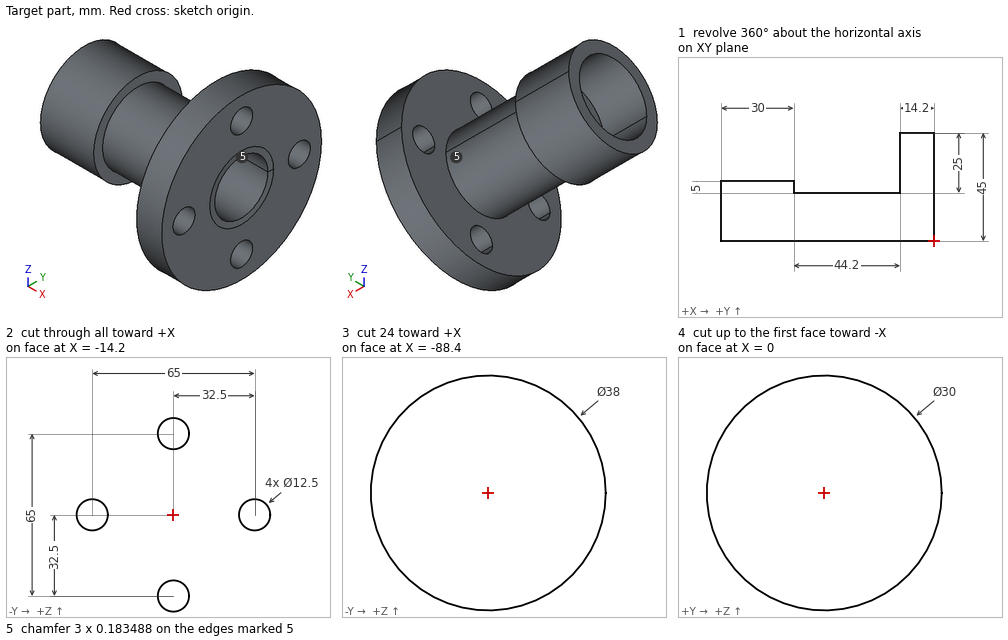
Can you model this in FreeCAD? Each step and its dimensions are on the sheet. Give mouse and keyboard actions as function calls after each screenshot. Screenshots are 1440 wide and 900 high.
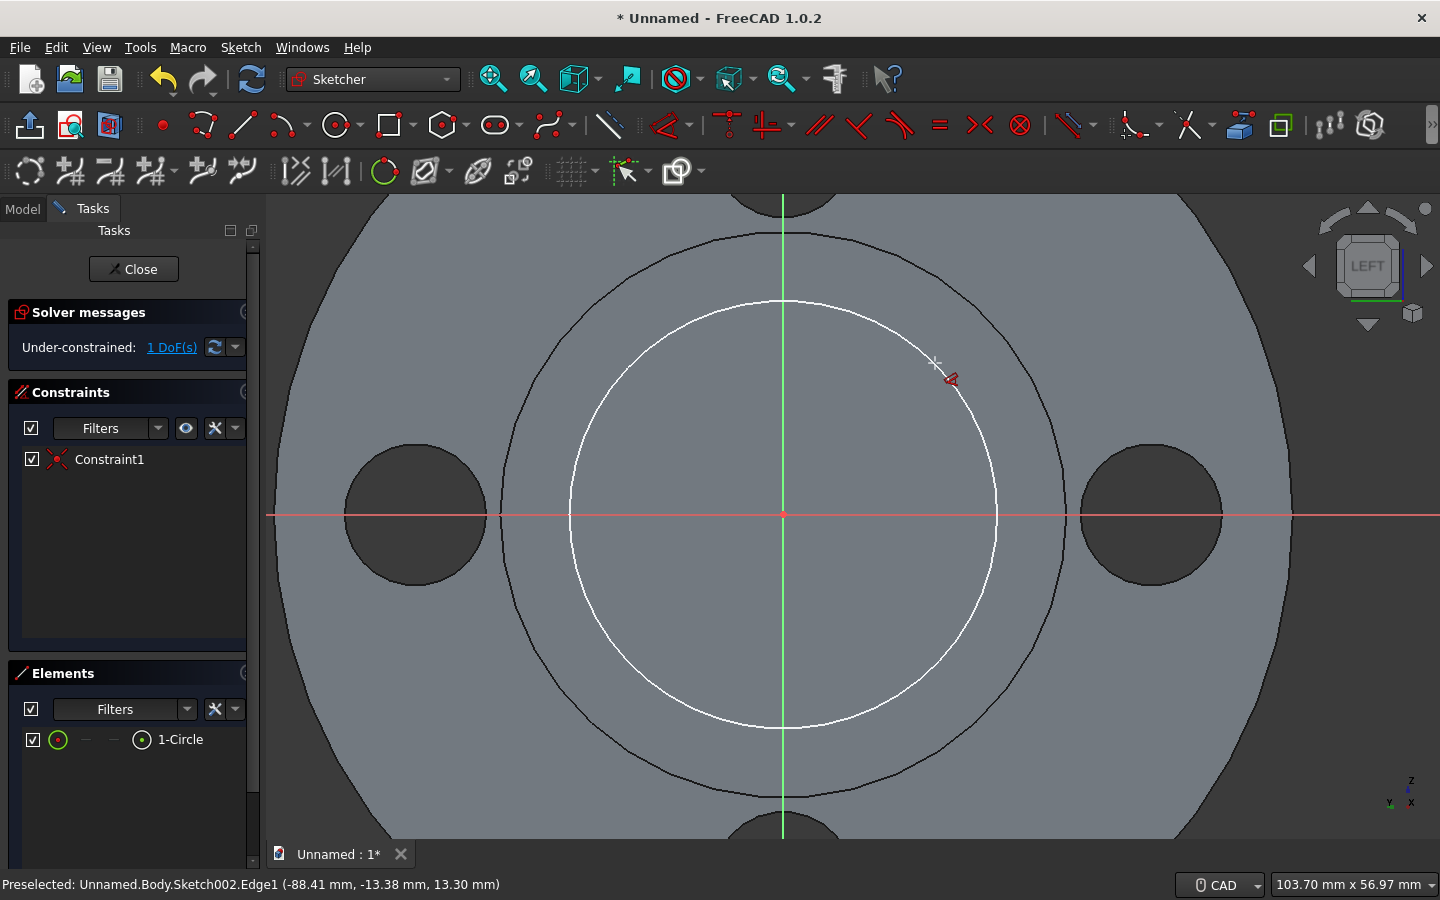
click(934, 363)
click(957, 340)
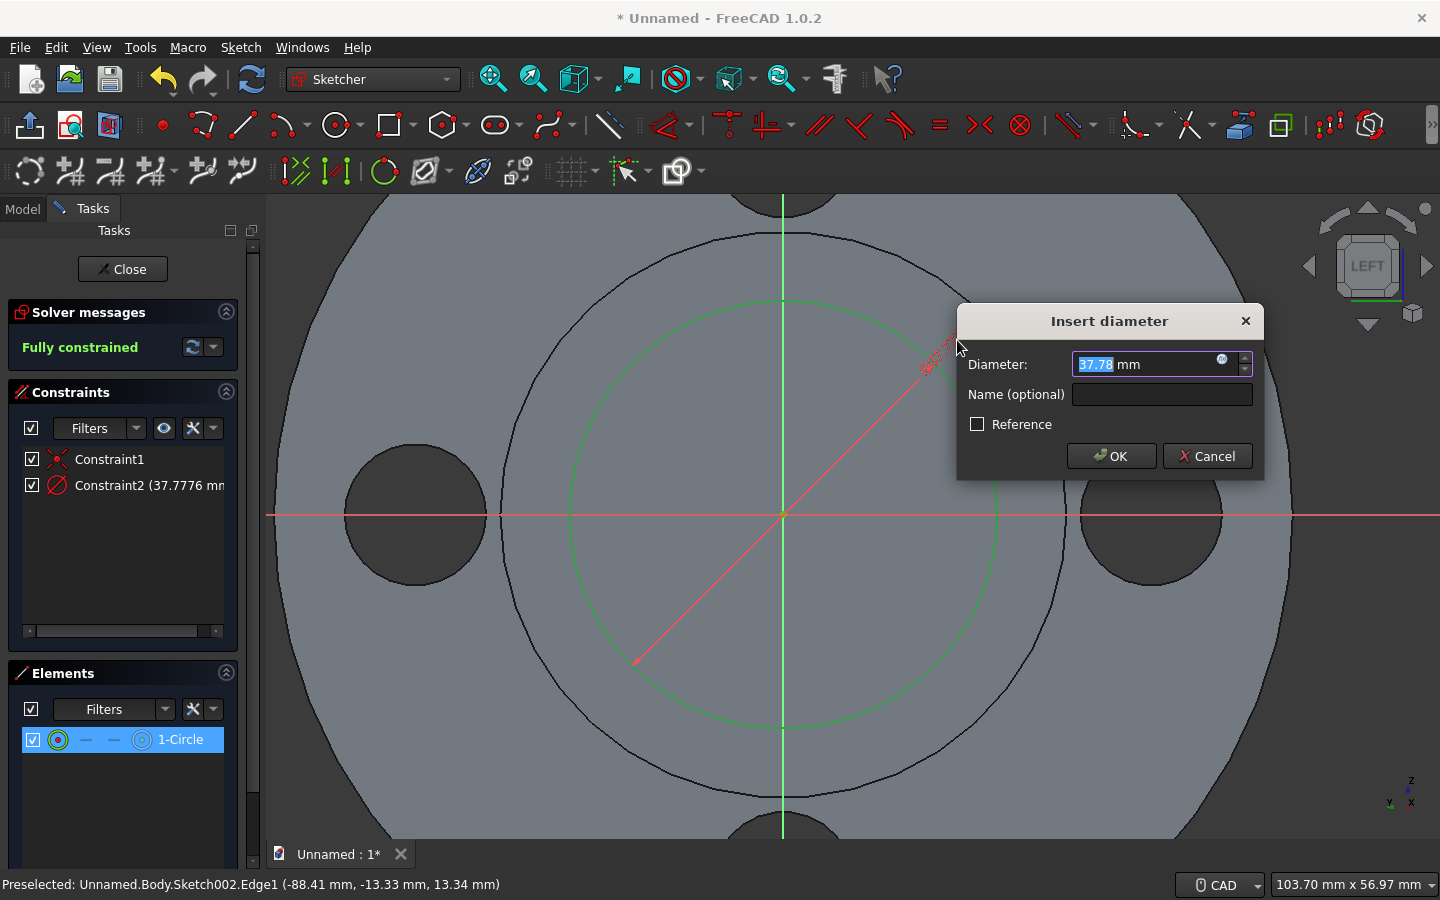
text(38)
key(Return)
key(Escape)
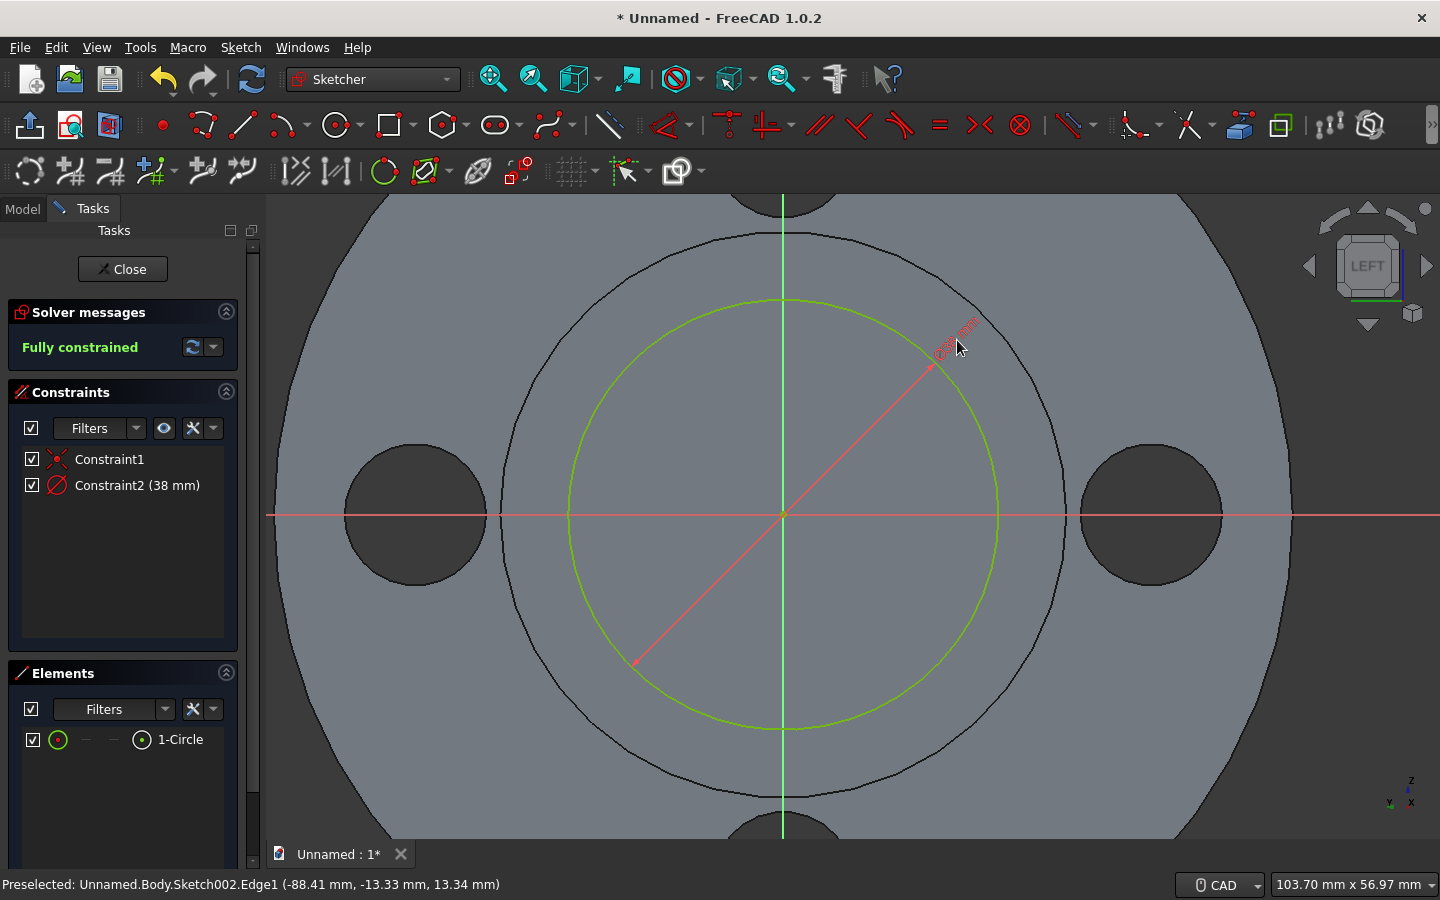
click(123, 269)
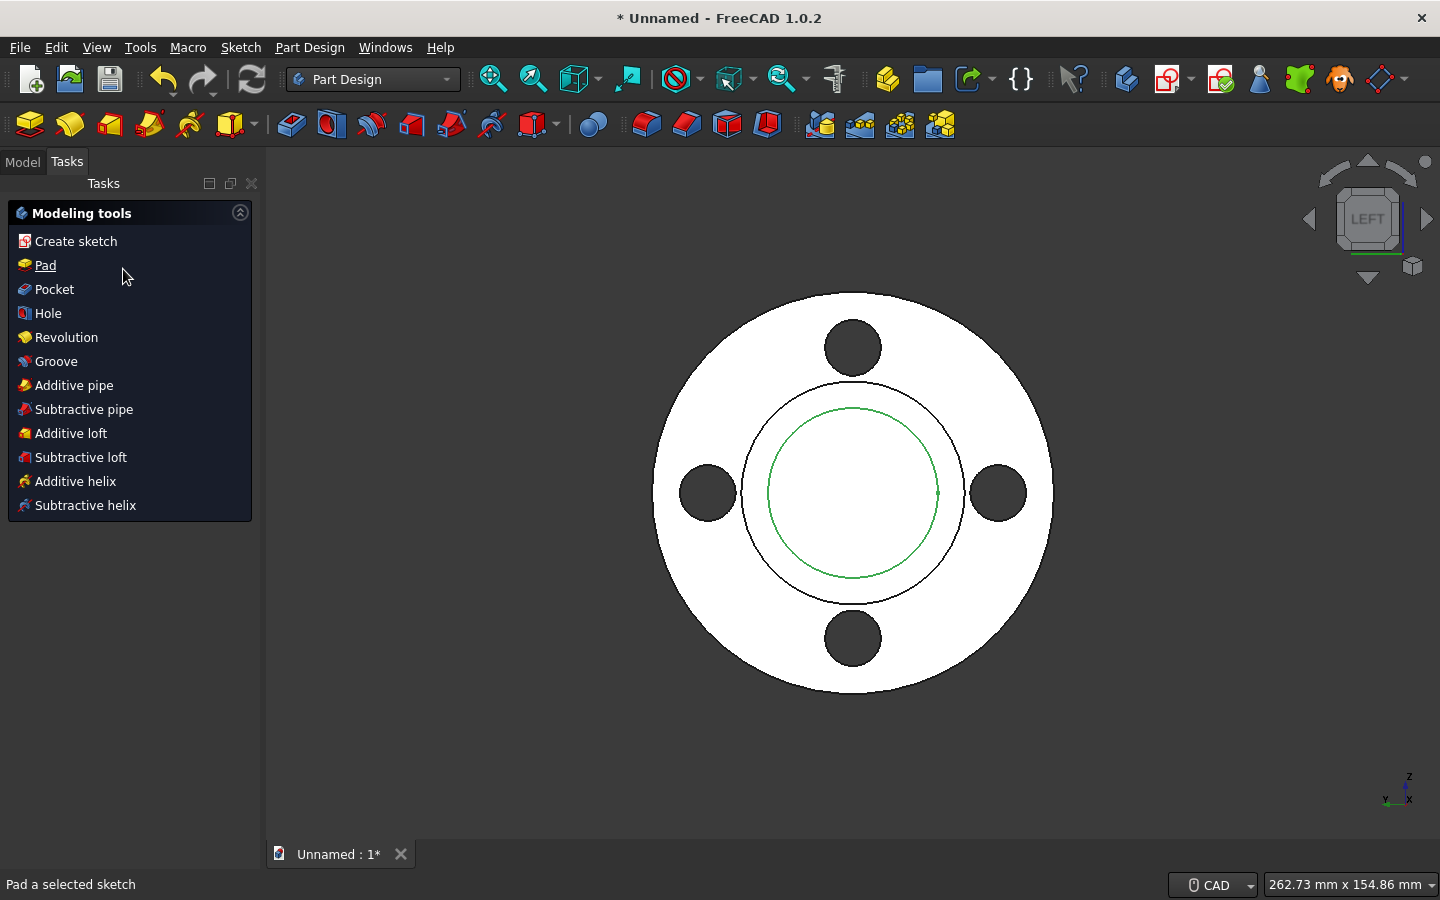
click(292, 124)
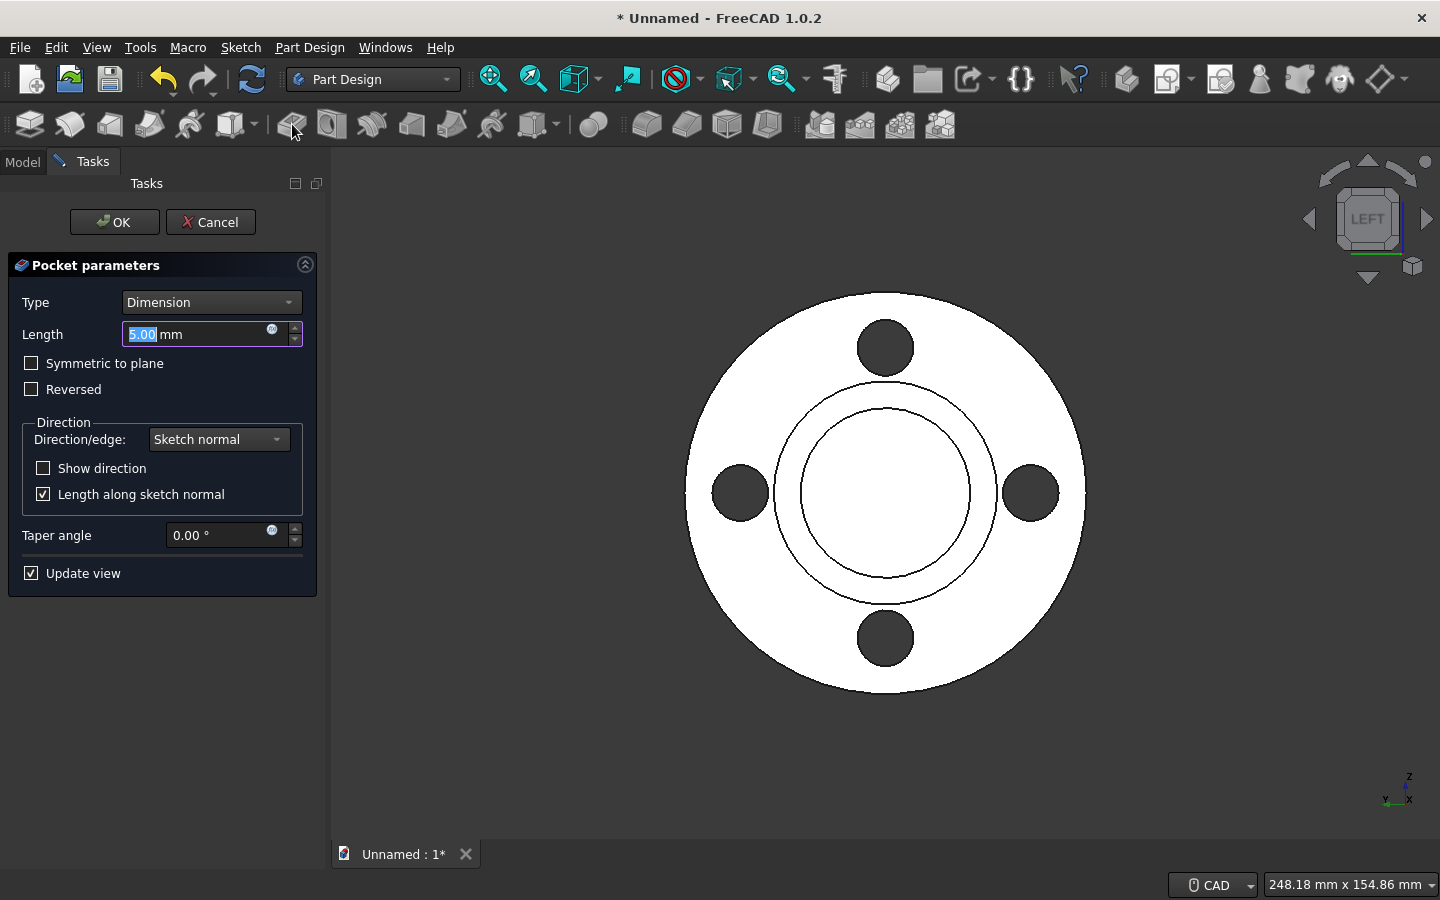
text(24)
key(Tab)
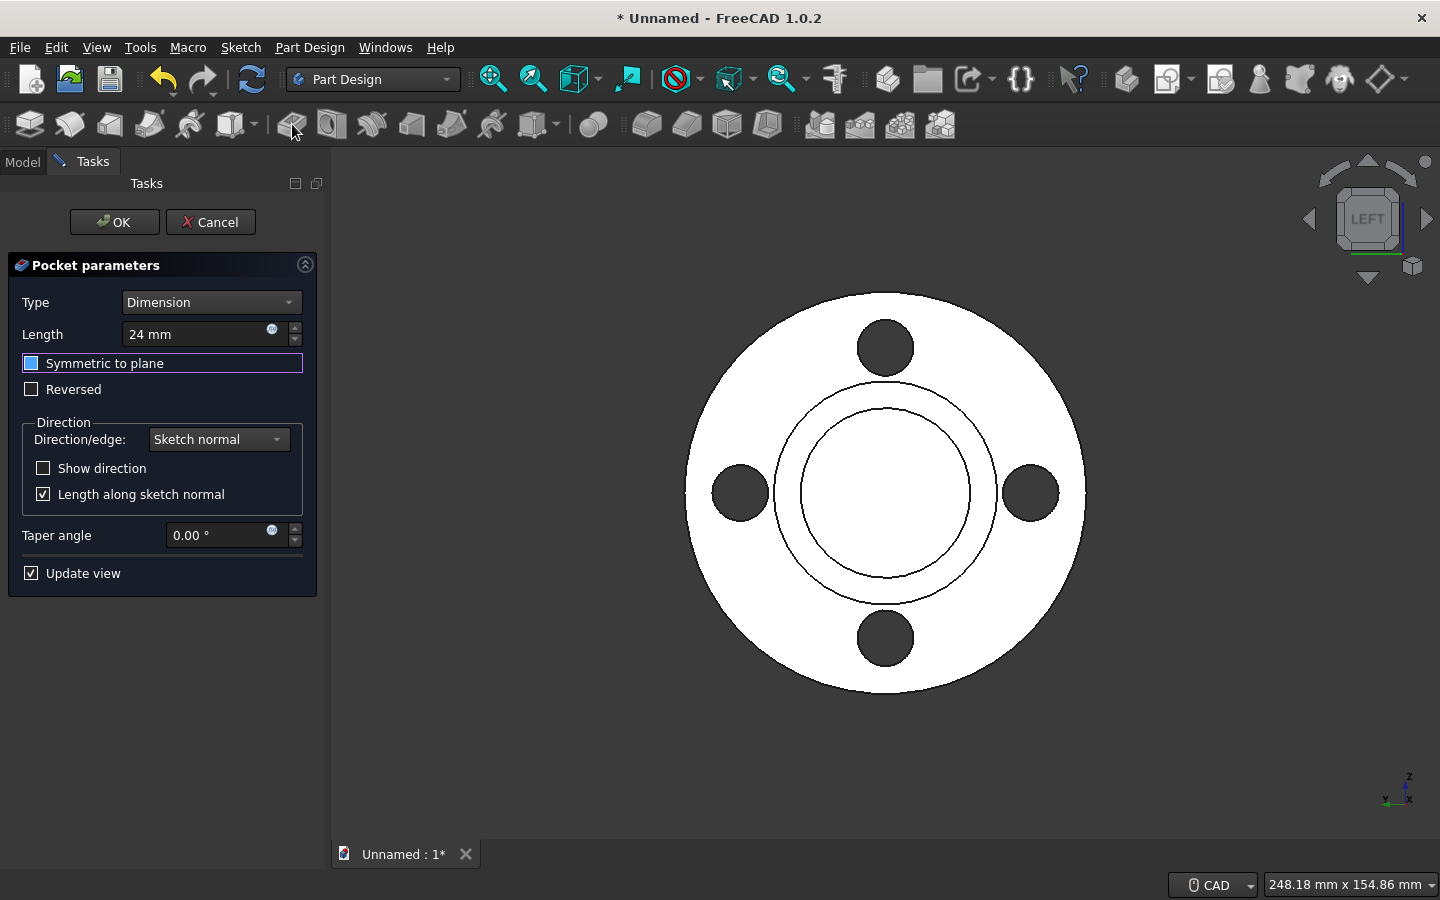
click(115, 222)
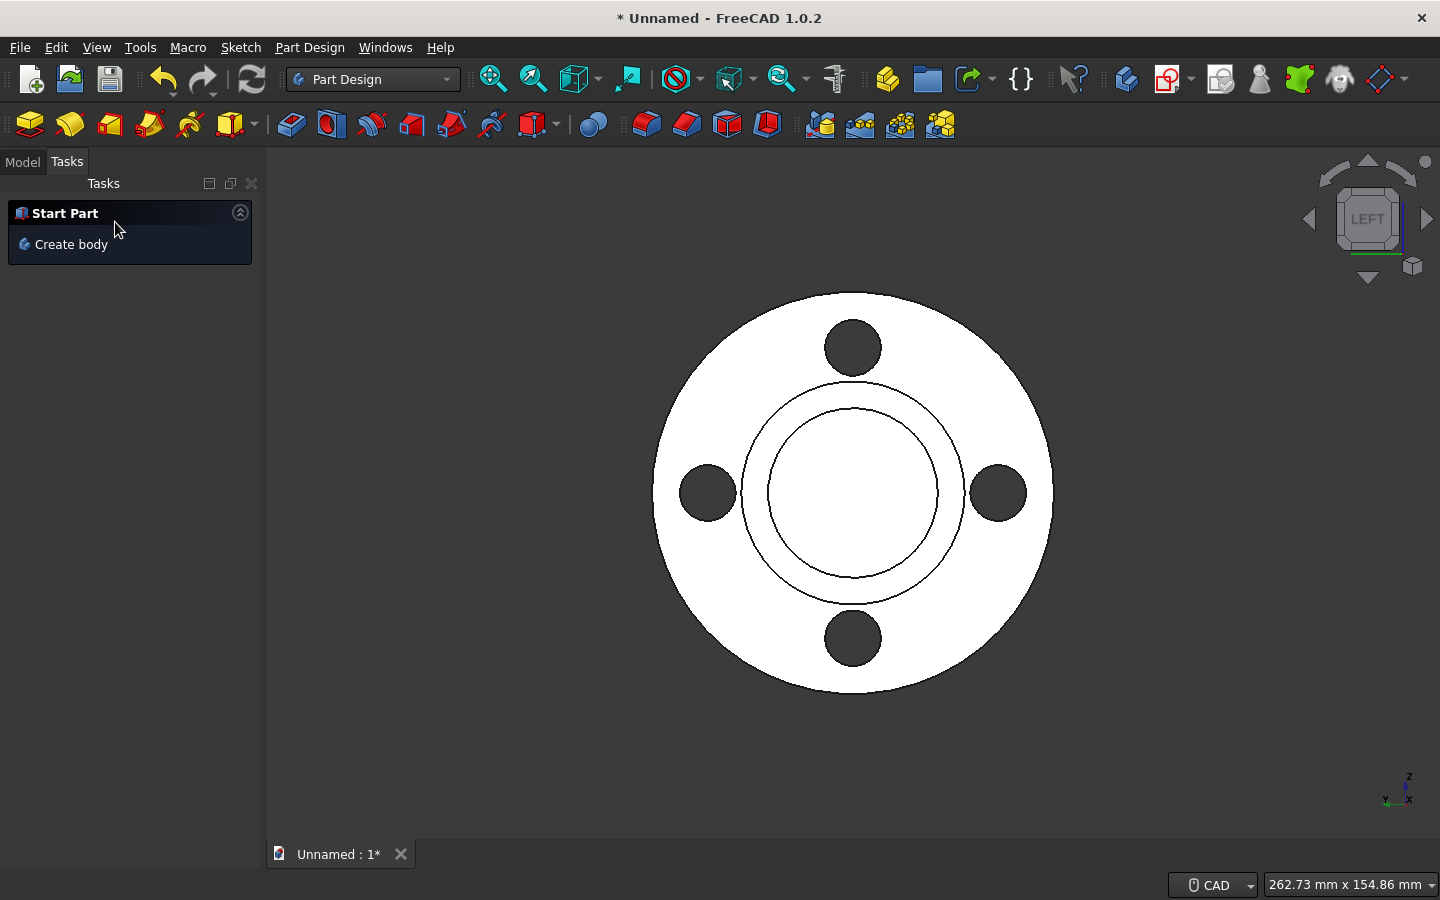
key(0)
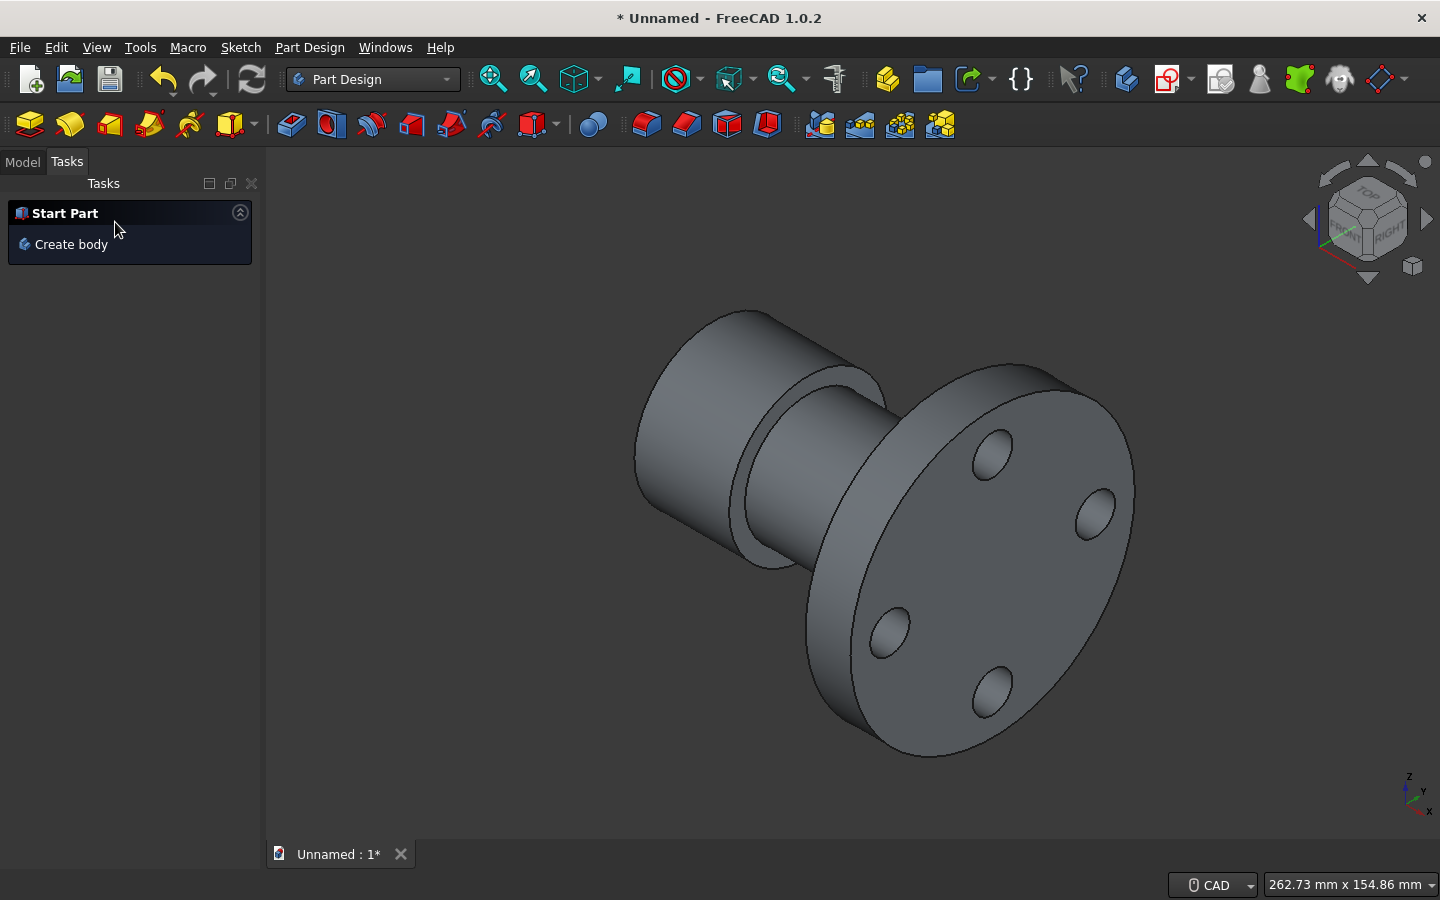
click(993, 573)